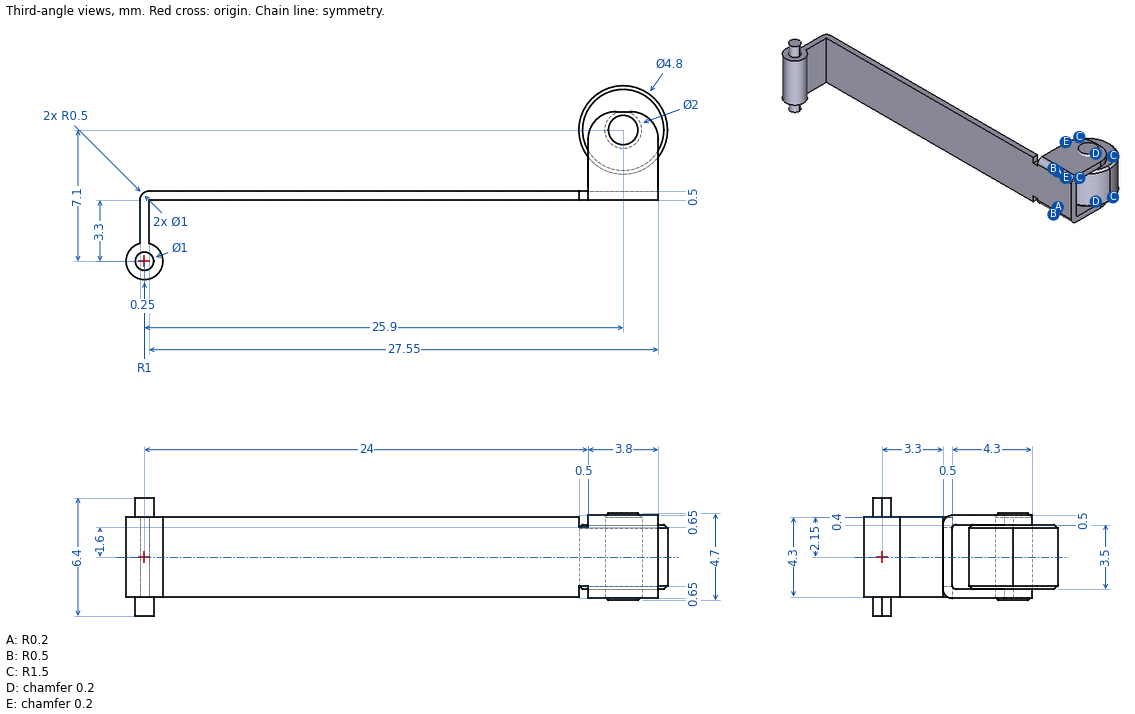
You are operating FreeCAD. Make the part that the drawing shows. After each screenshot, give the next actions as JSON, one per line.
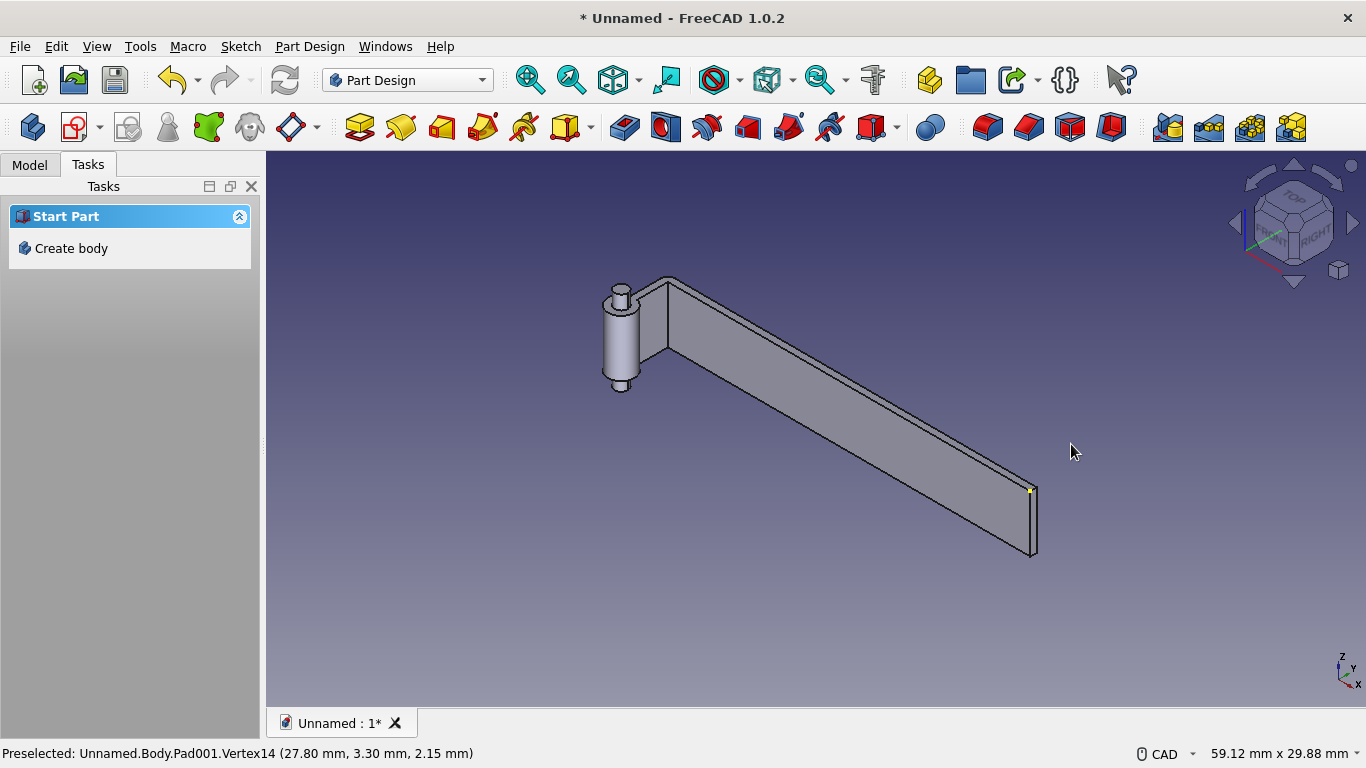
{"action": "scroll", "coordinate": [1034, 493], "scroll_direction": "up", "scroll_amount": 5}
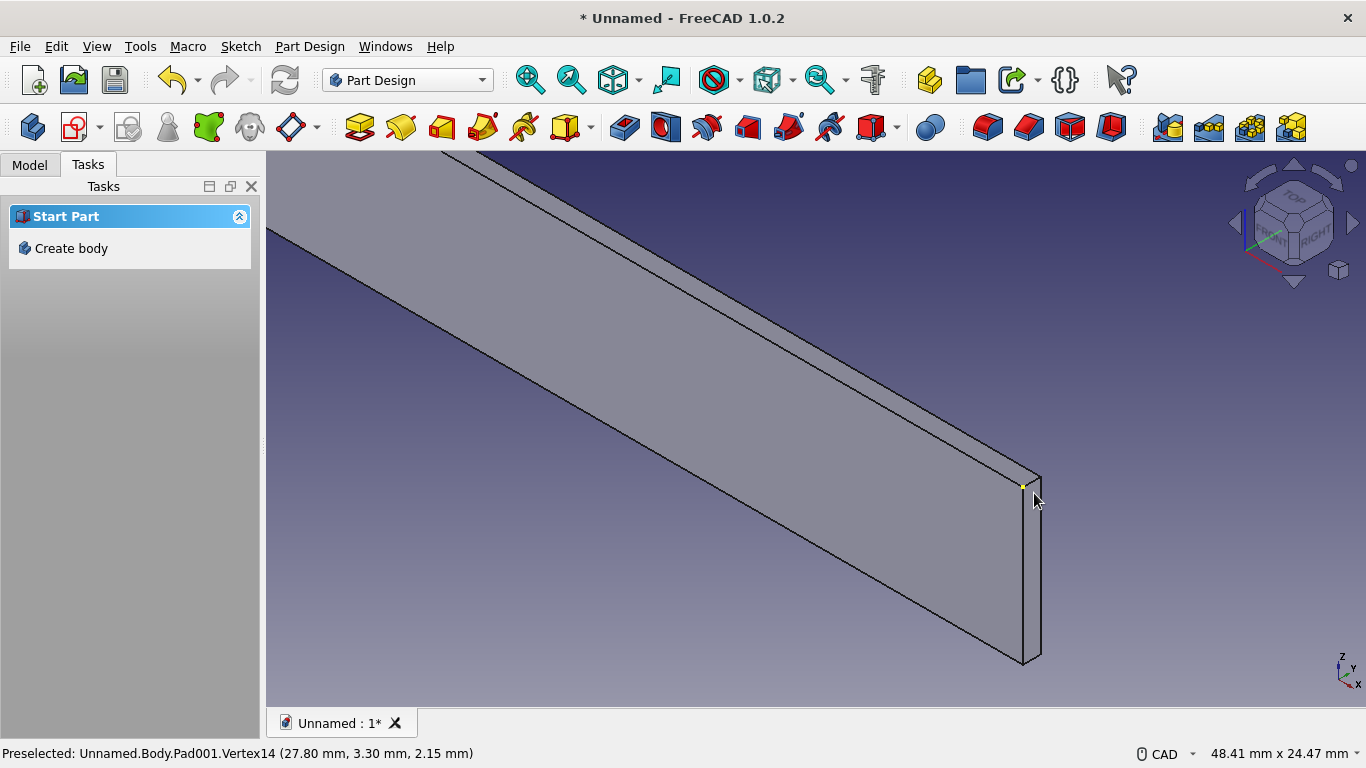
{"action": "left_click", "coordinate": [1032, 494]}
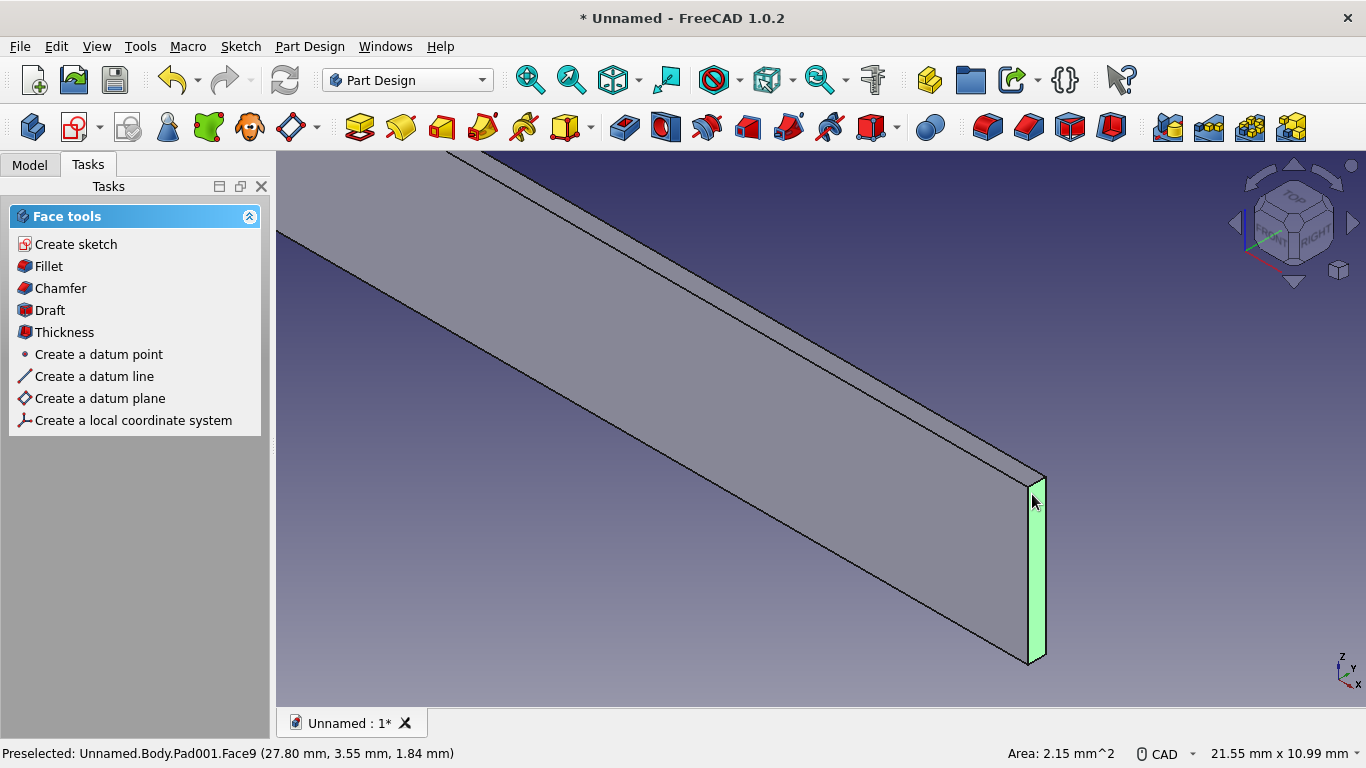
{"action": "left_click", "coordinate": [74, 128]}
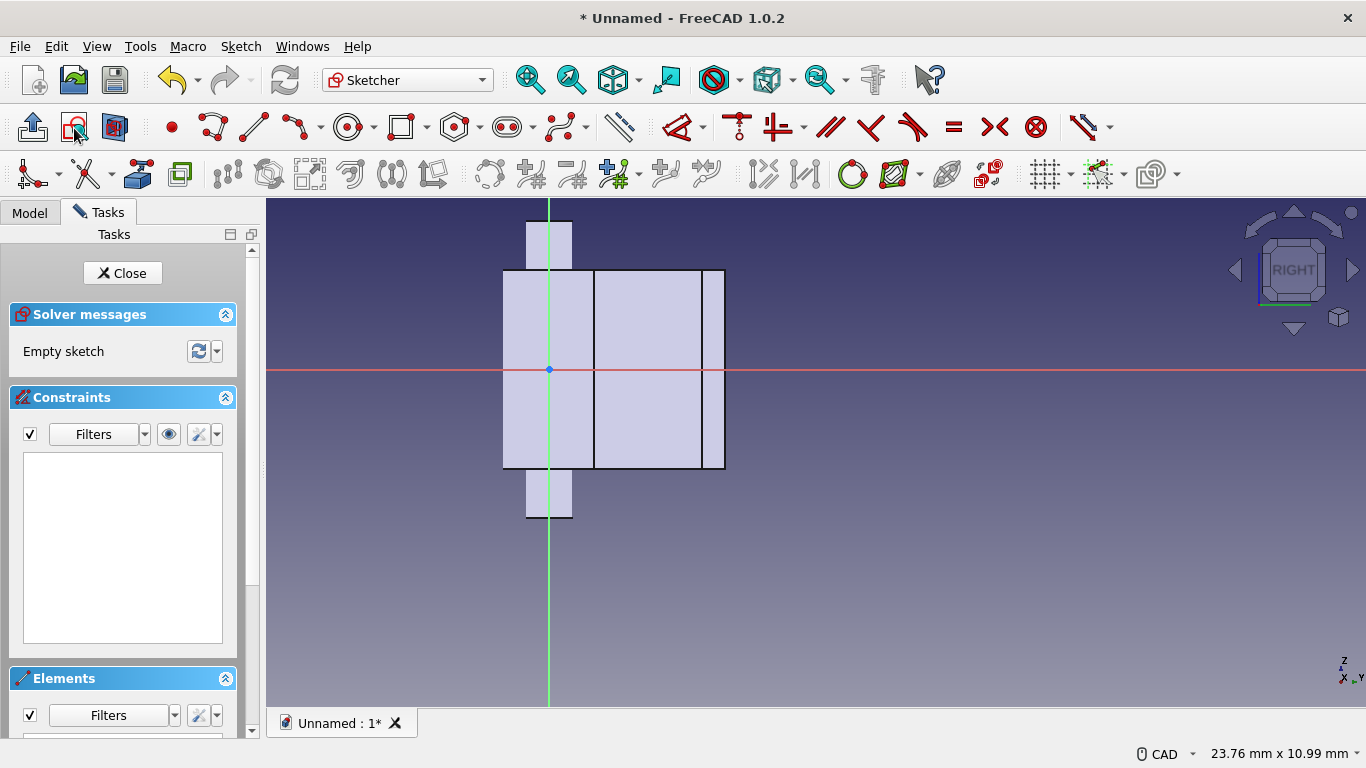
{"action": "scroll", "coordinate": [715, 226], "scroll_direction": "up", "scroll_amount": 2}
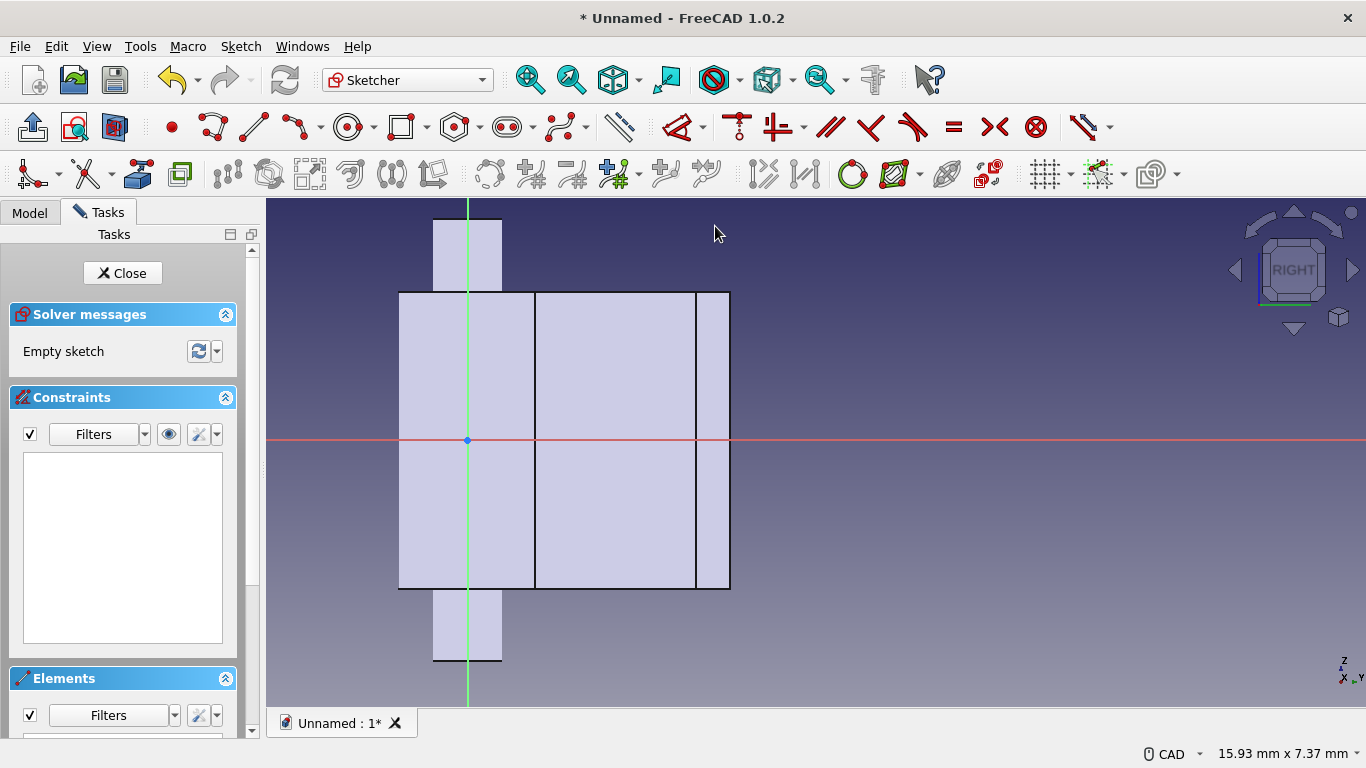
{"action": "key", "text": "g m"}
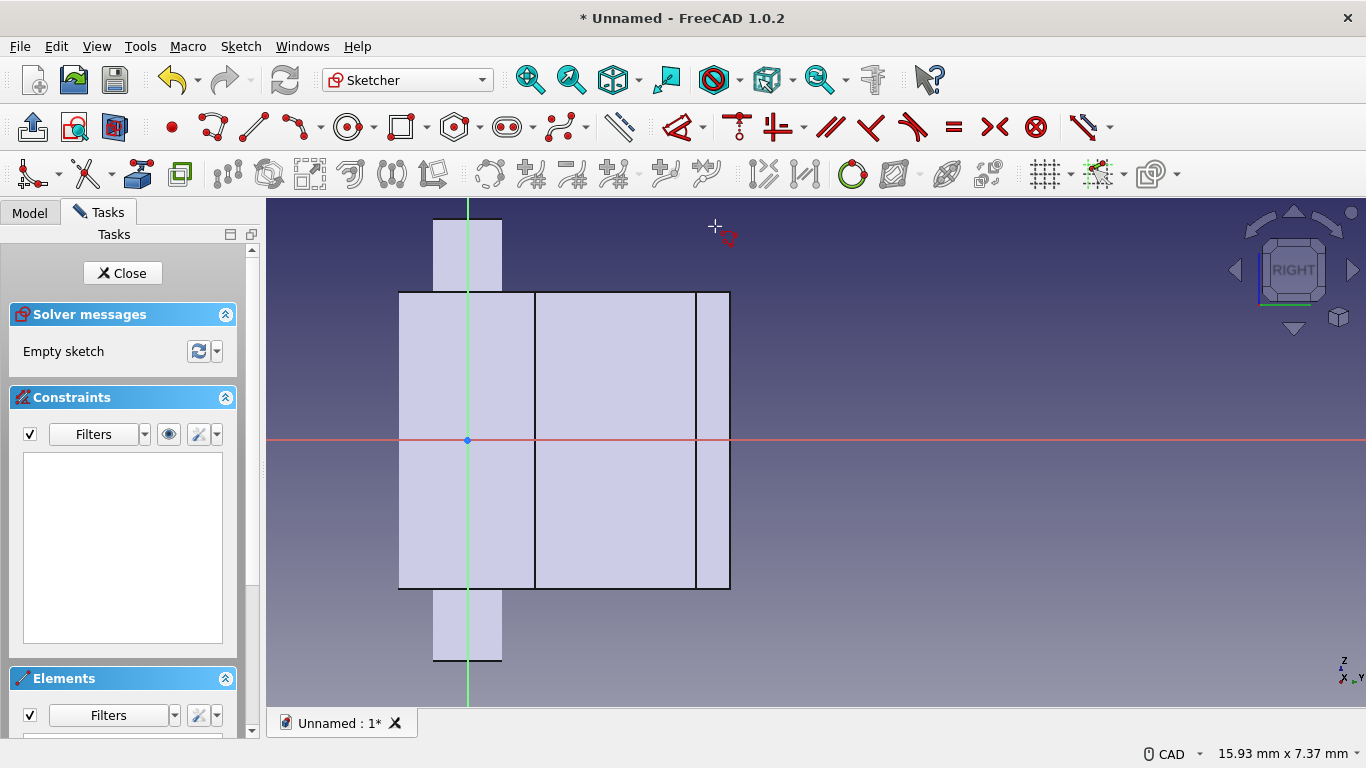
{"action": "left_click", "coordinate": [696, 292]}
{"action": "left_click", "coordinate": [730, 292]}
{"action": "left_click", "coordinate": [730, 319]}
{"action": "left_click", "coordinate": [1027, 319]}
{"action": "left_click", "coordinate": [1027, 285]}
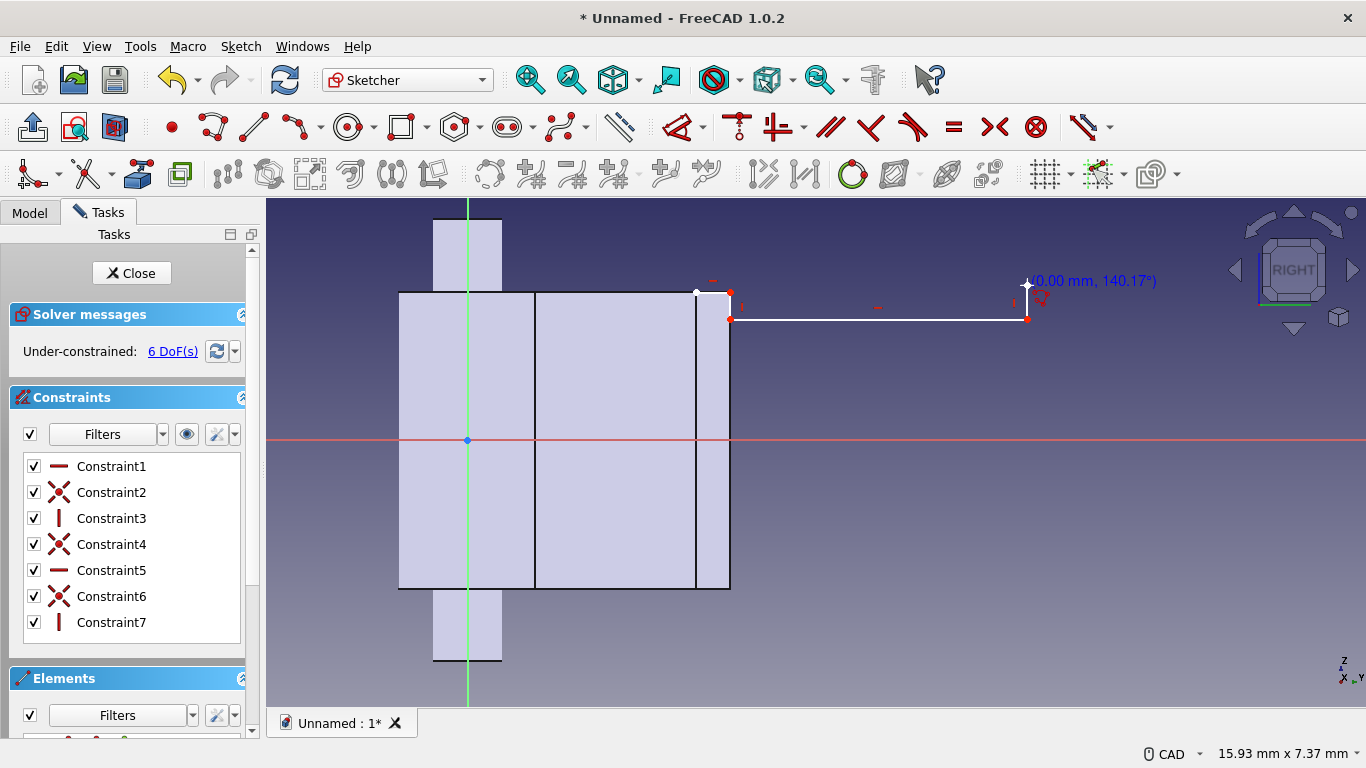
{"action": "scroll", "coordinate": [696, 285], "scroll_direction": "up", "scroll_amount": 5}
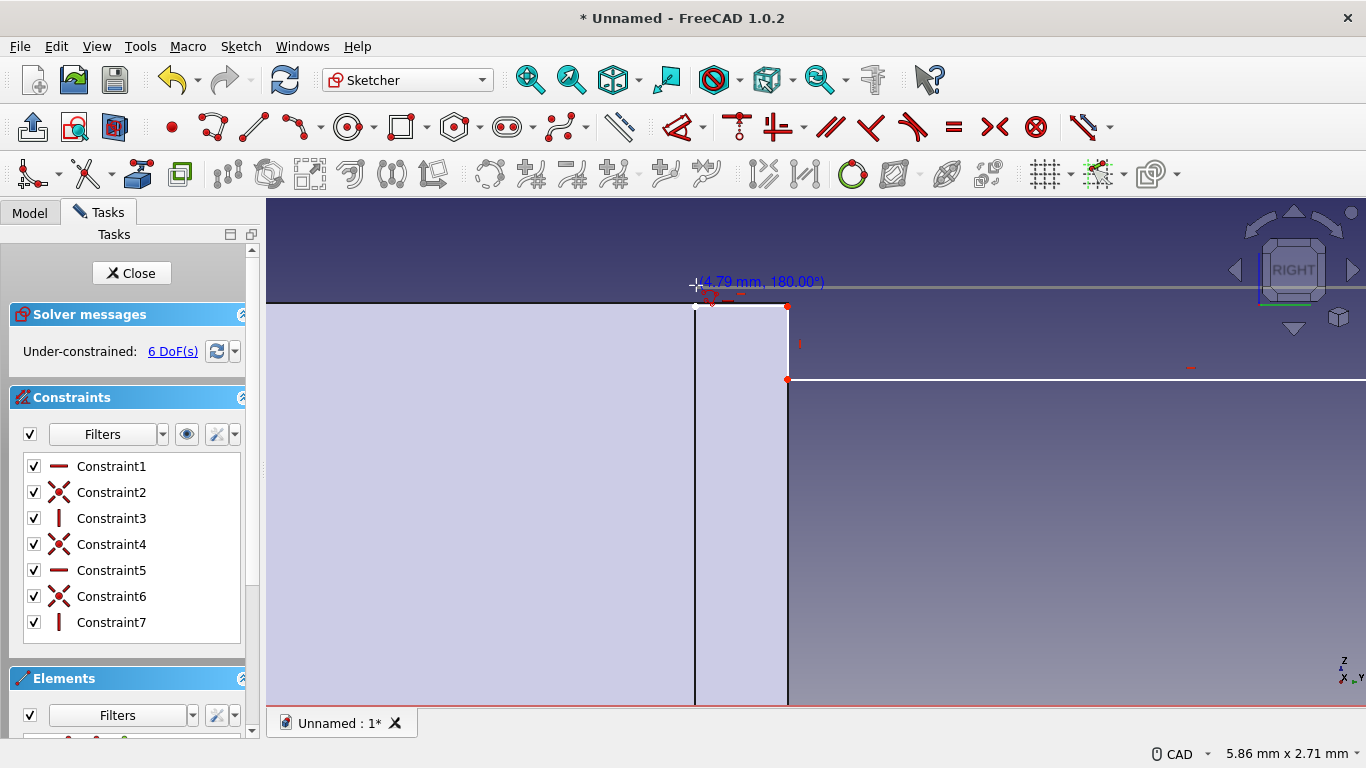
{"action": "left_click", "coordinate": [695, 285]}
{"action": "left_click", "coordinate": [695, 306]}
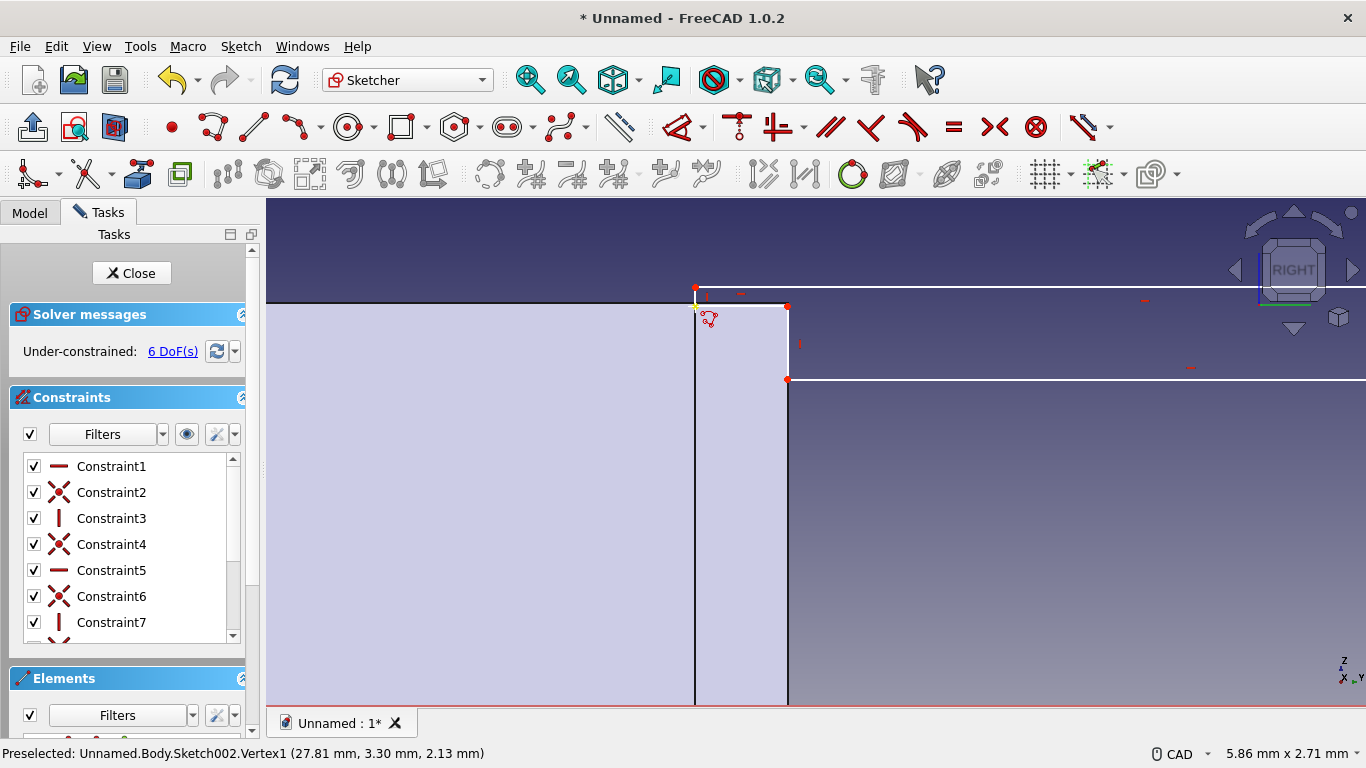
{"action": "scroll", "coordinate": [696, 305], "scroll_direction": "down", "scroll_amount": 5}